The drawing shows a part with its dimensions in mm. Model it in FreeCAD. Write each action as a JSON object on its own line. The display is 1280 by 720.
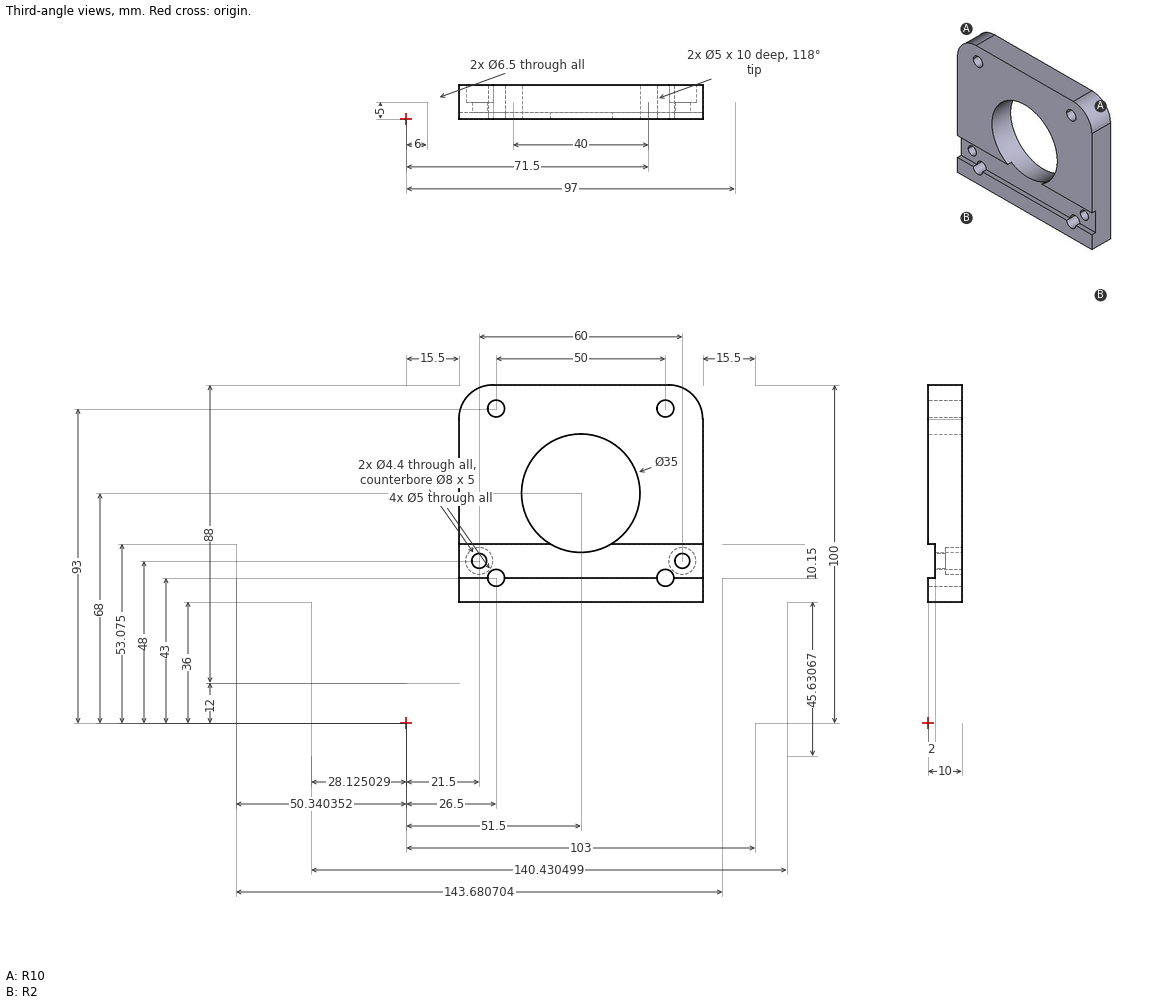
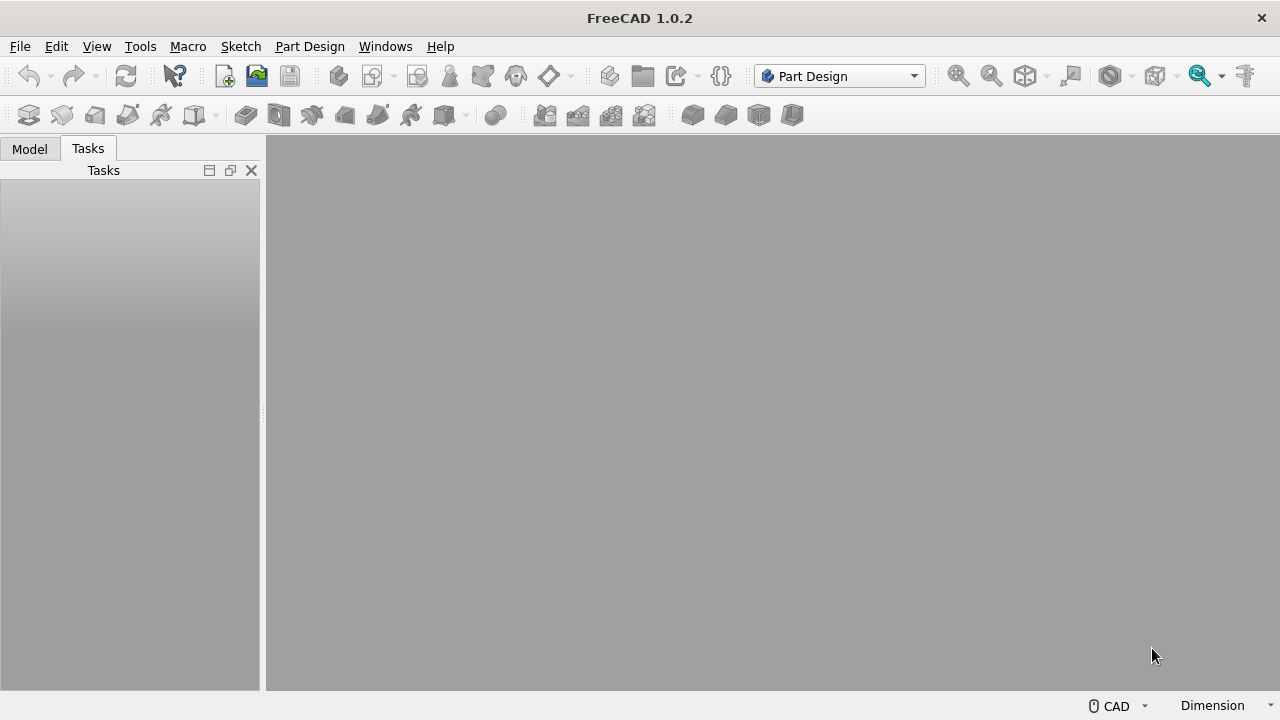
{"action": "key", "text": "ctrl+n"}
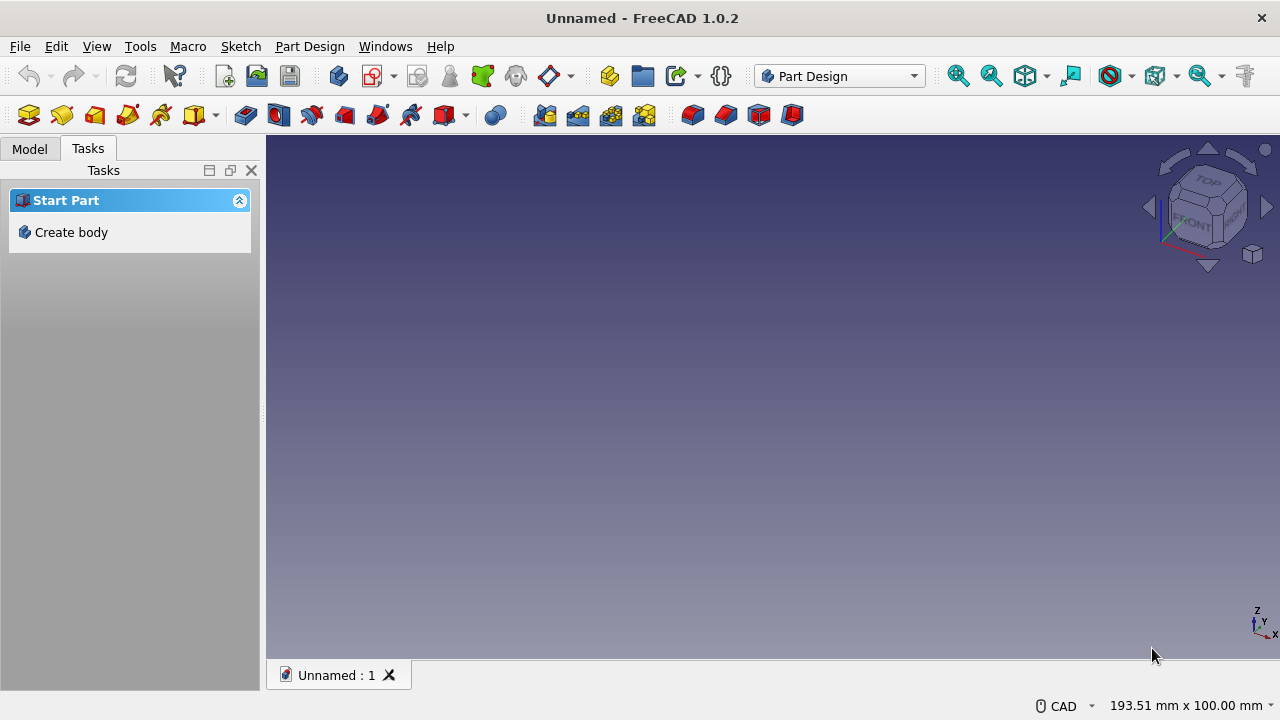
{"action": "left_click", "coordinate": [372, 76]}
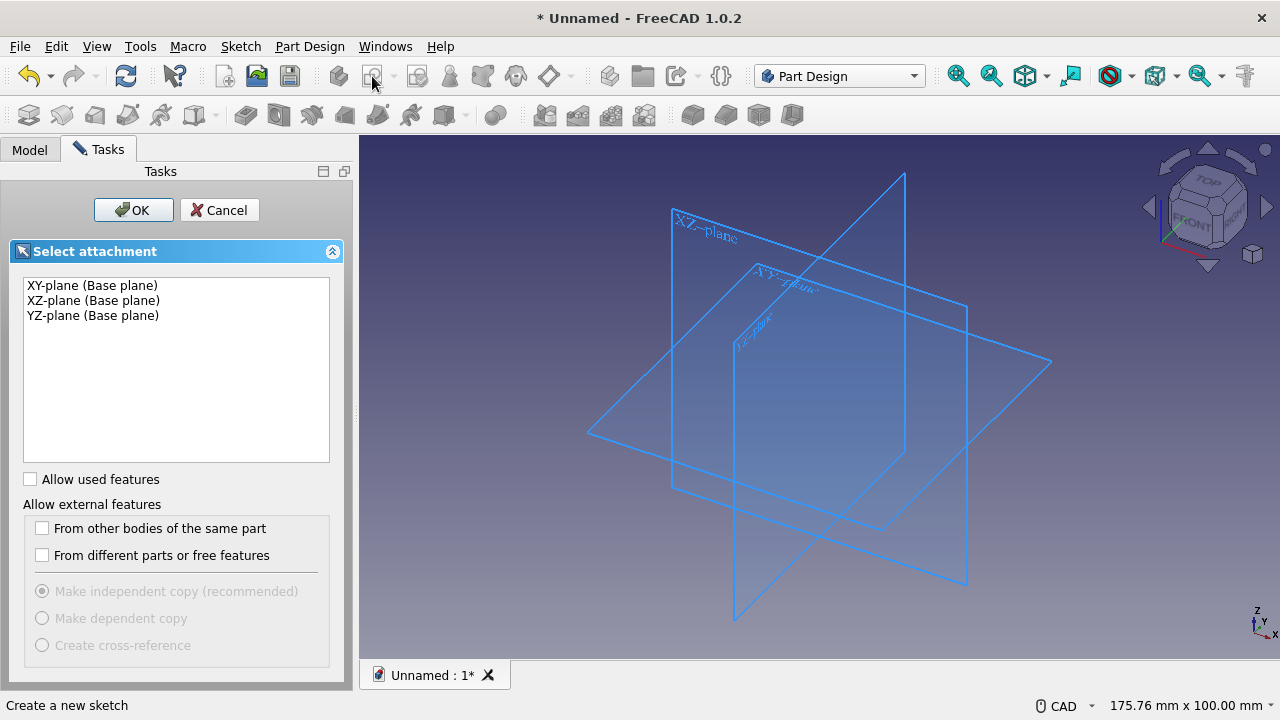
{"action": "left_click", "coordinate": [84, 300]}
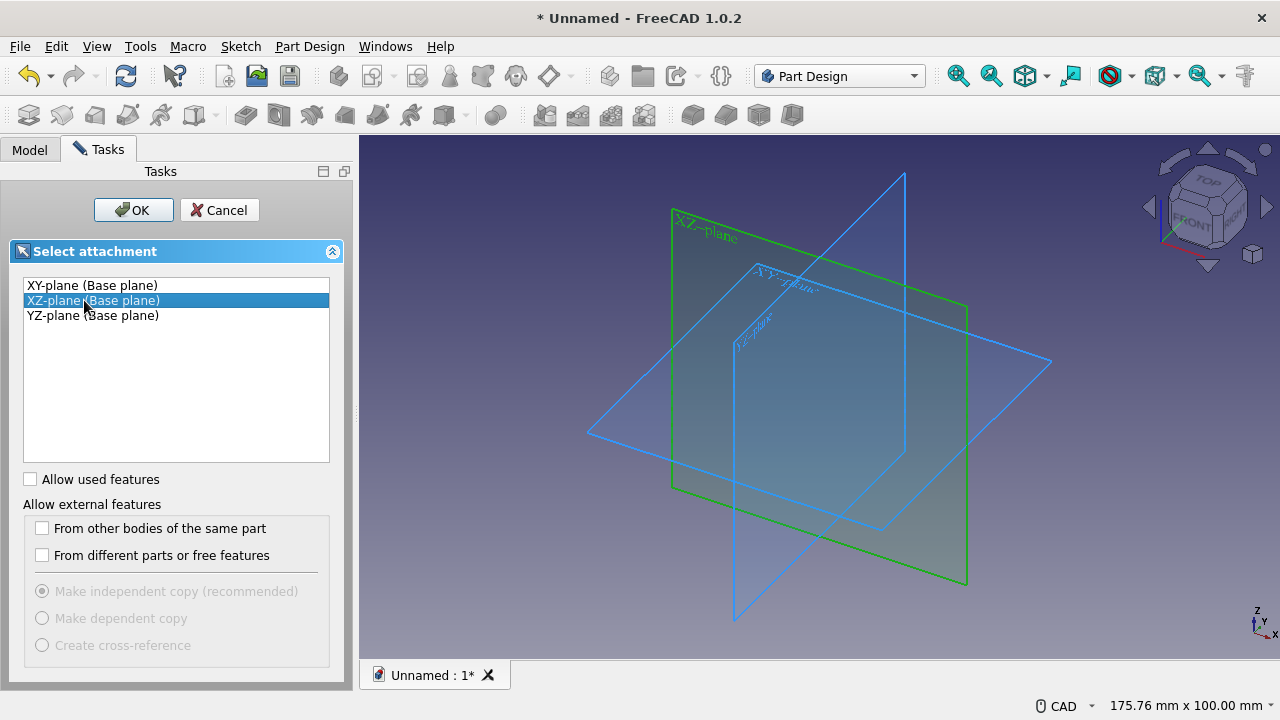
{"action": "left_click", "coordinate": [134, 210]}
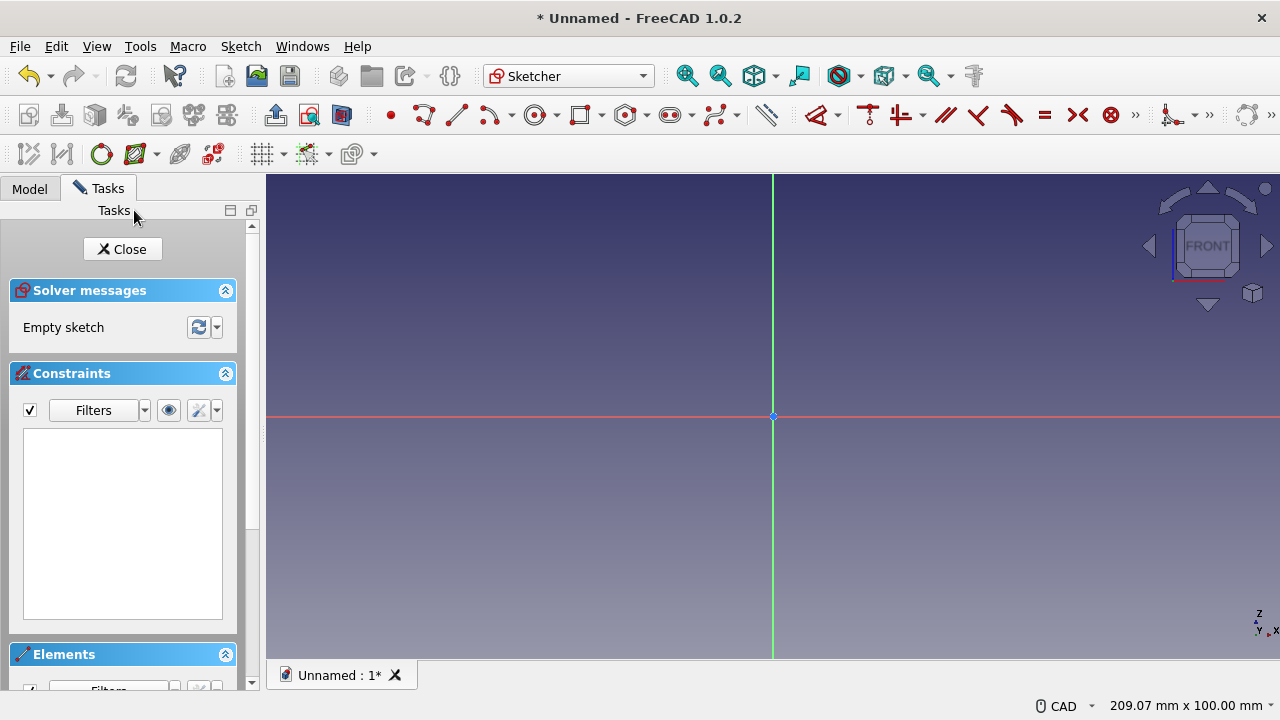
{"action": "scroll", "coordinate": [317, 631], "scroll_direction": "down", "scroll_amount": 3}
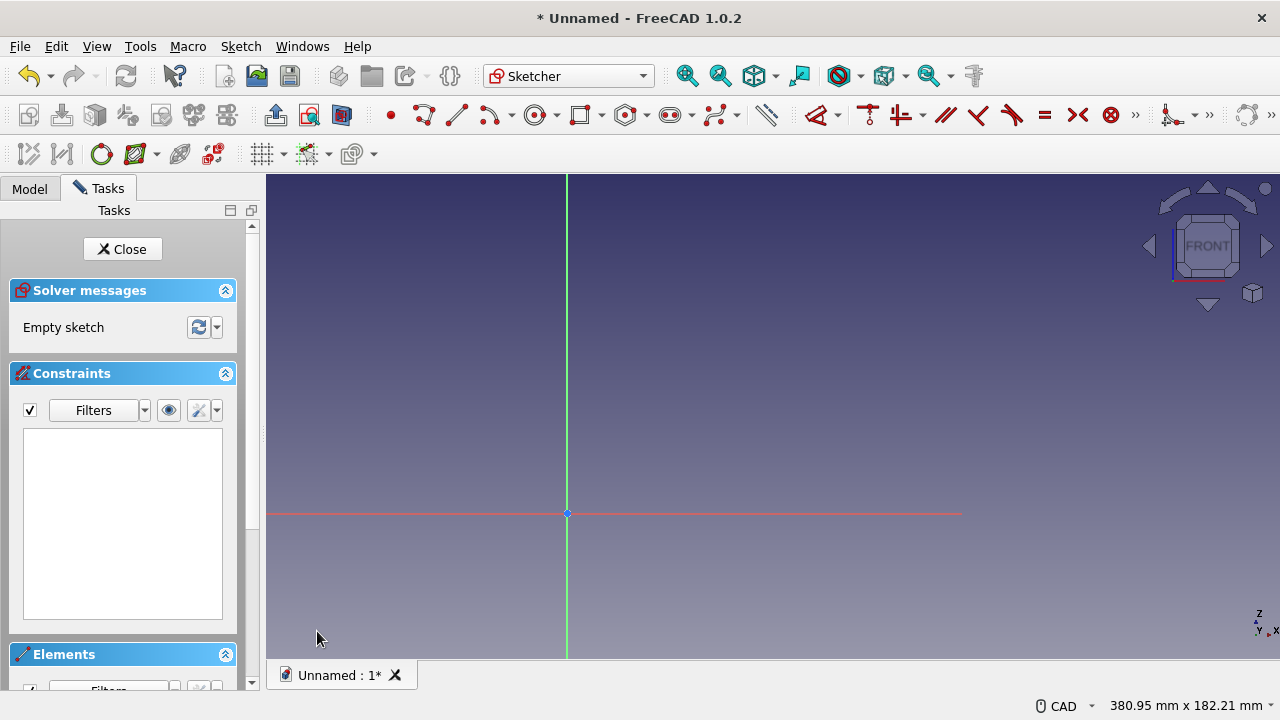
{"action": "key", "text": "g r"}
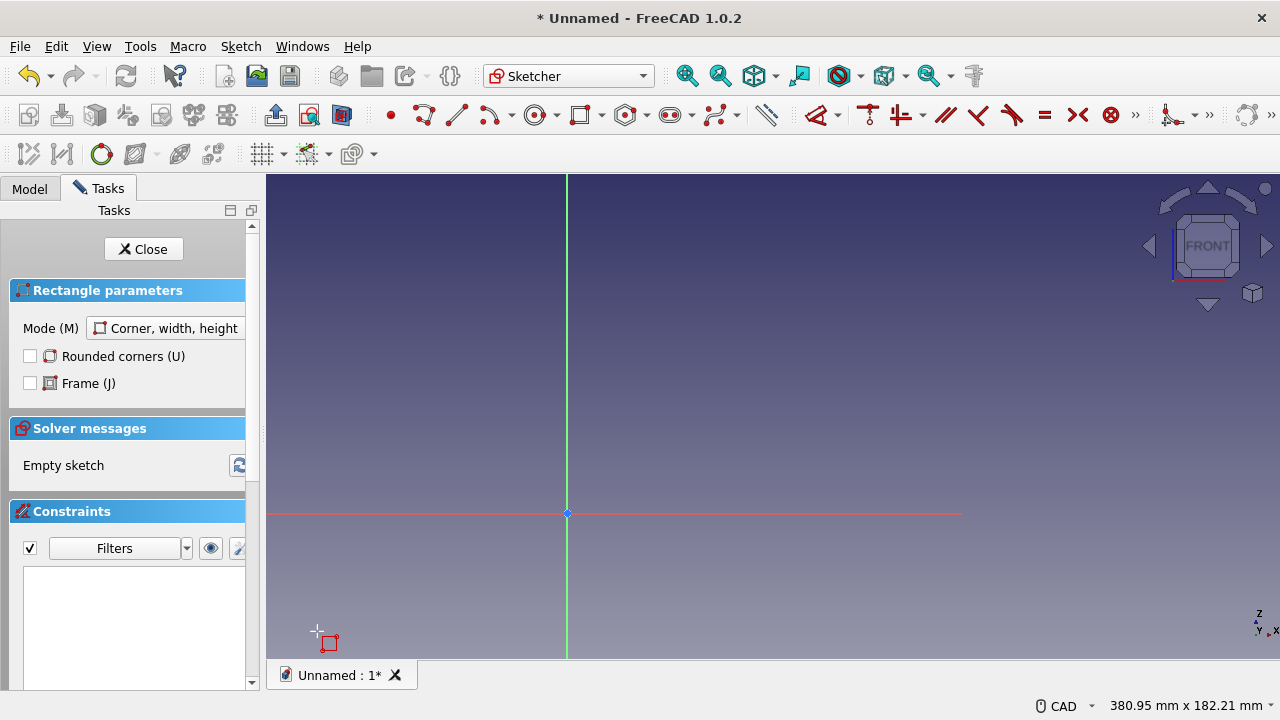
{"action": "left_click", "coordinate": [567, 514]}
{"action": "mouse_move", "coordinate": [841, 248]}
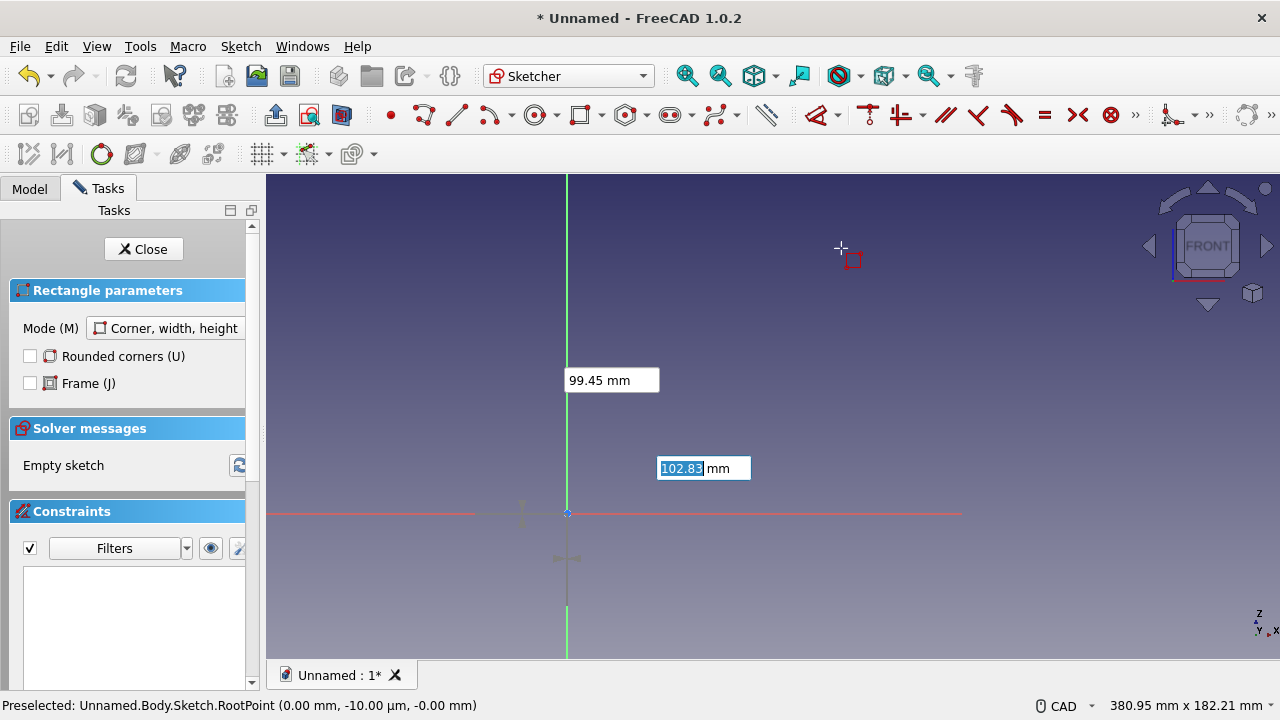
{"action": "type", "text": "103"}
{"action": "key", "text": "Tab"}
{"action": "type", "text": "100"}
{"action": "key", "text": "Return"}
{"action": "key", "text": "Escape"}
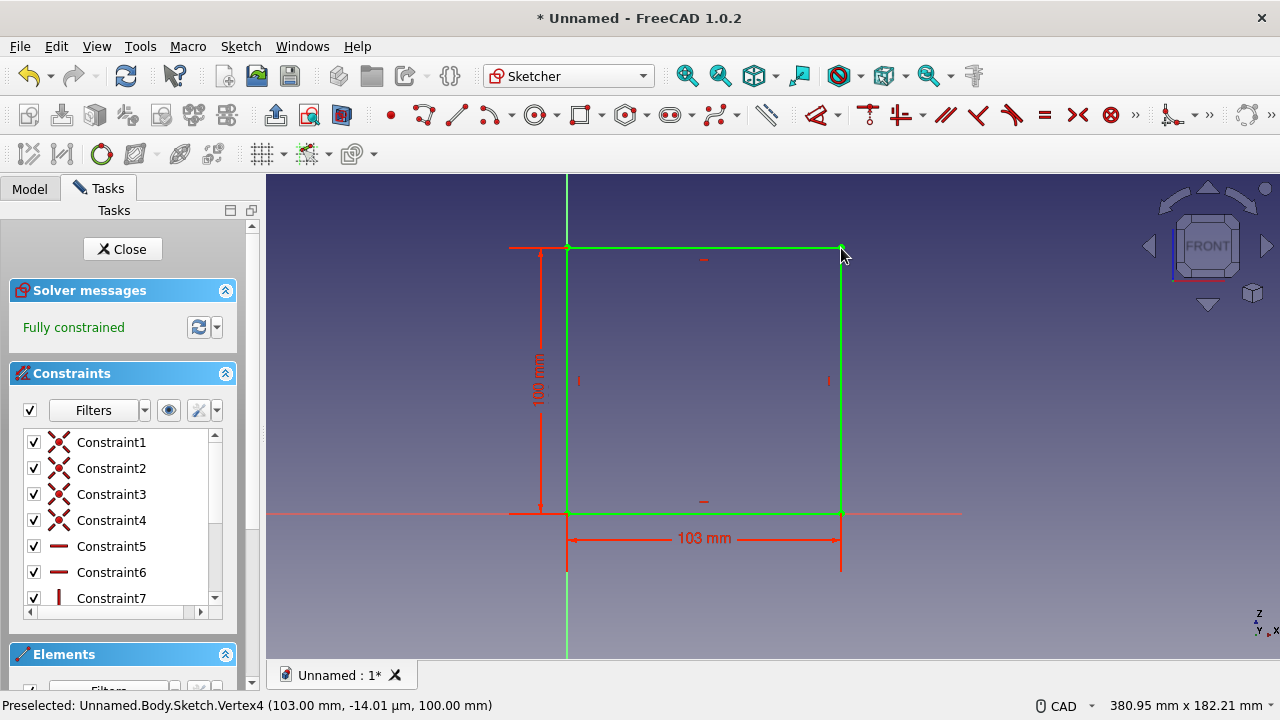
{"action": "left_click", "coordinate": [123, 249]}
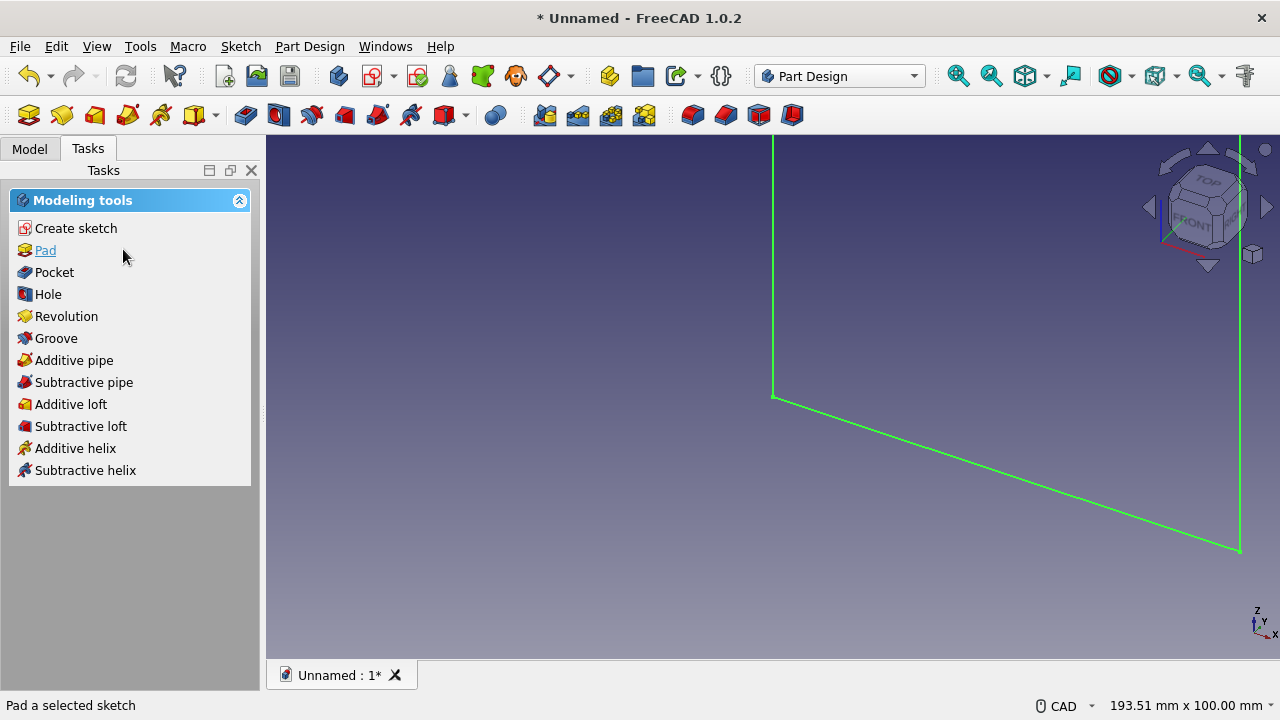
{"action": "left_click", "coordinate": [29, 116]}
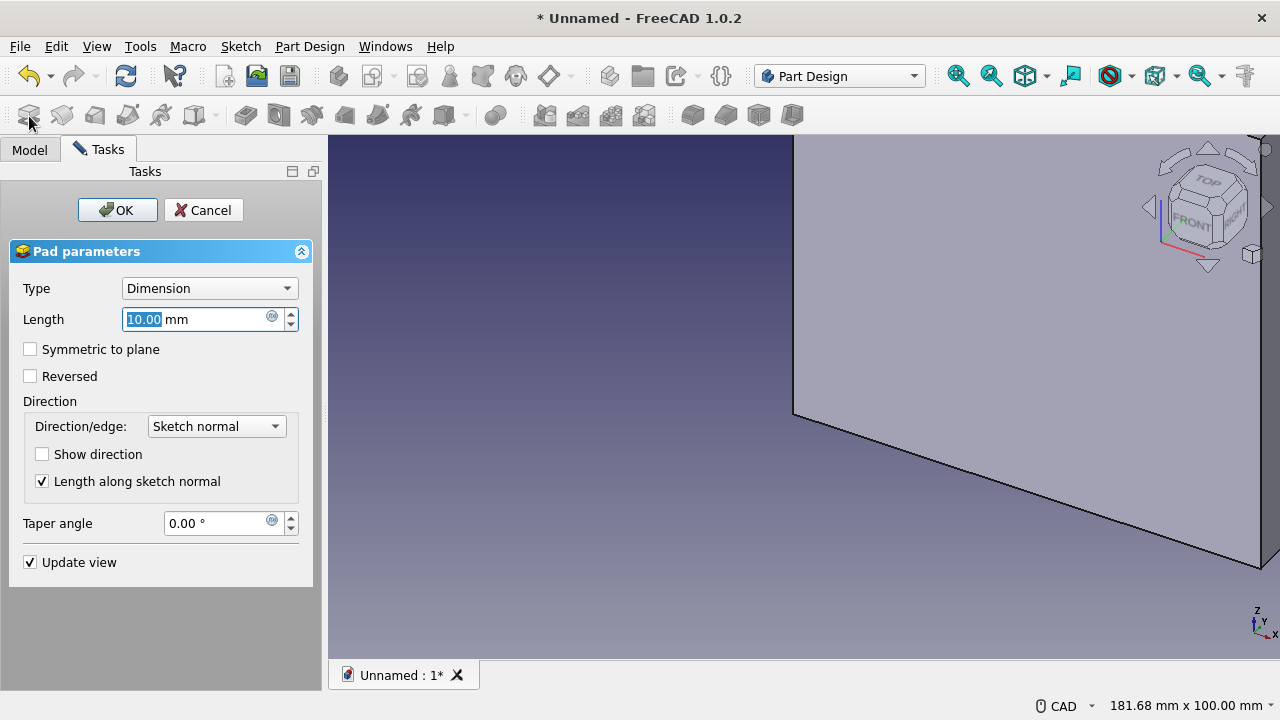
{"action": "type", "text": "10"}
{"action": "key", "text": "Tab"}